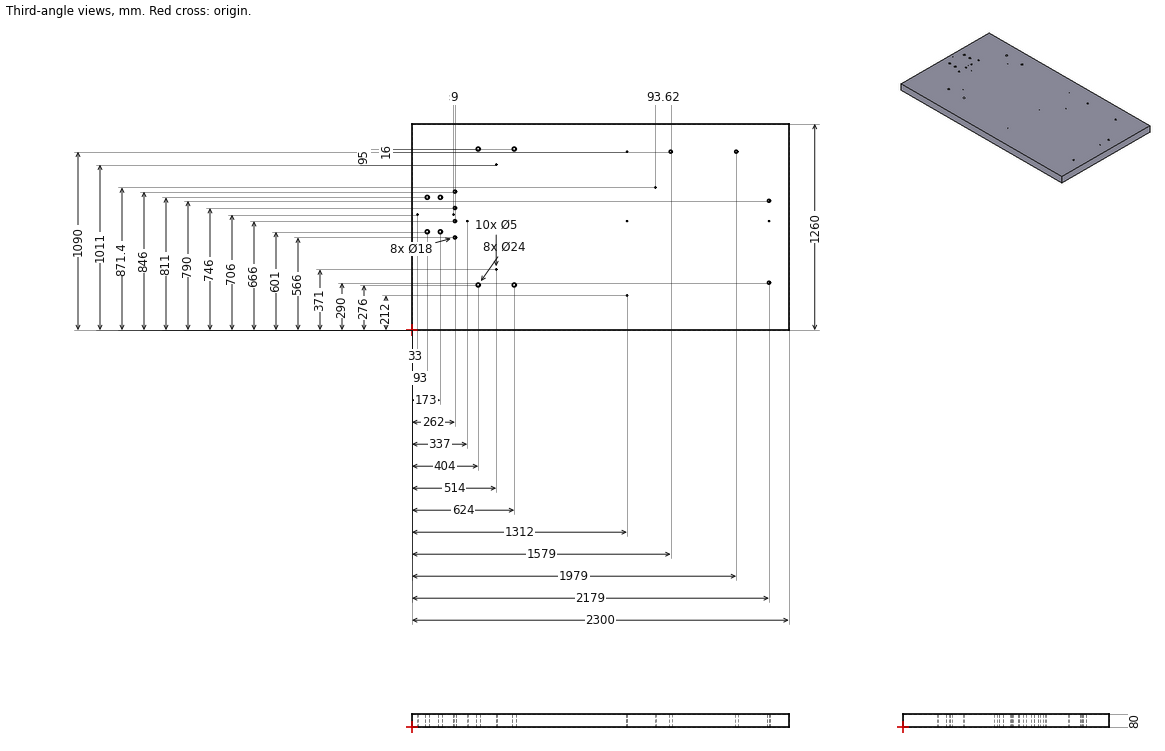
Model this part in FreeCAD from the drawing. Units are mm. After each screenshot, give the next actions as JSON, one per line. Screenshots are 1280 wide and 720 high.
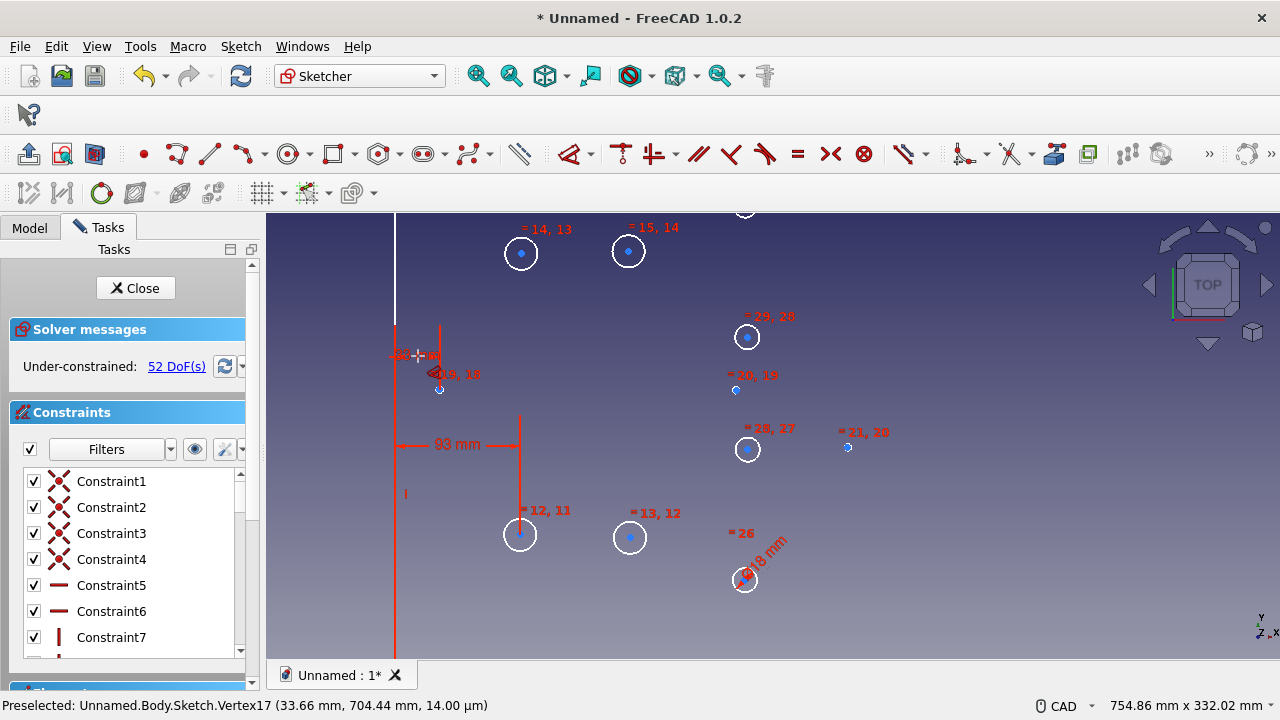
{"action": "scroll", "coordinate": [460, 425], "scroll_direction": "down", "scroll_amount": 9}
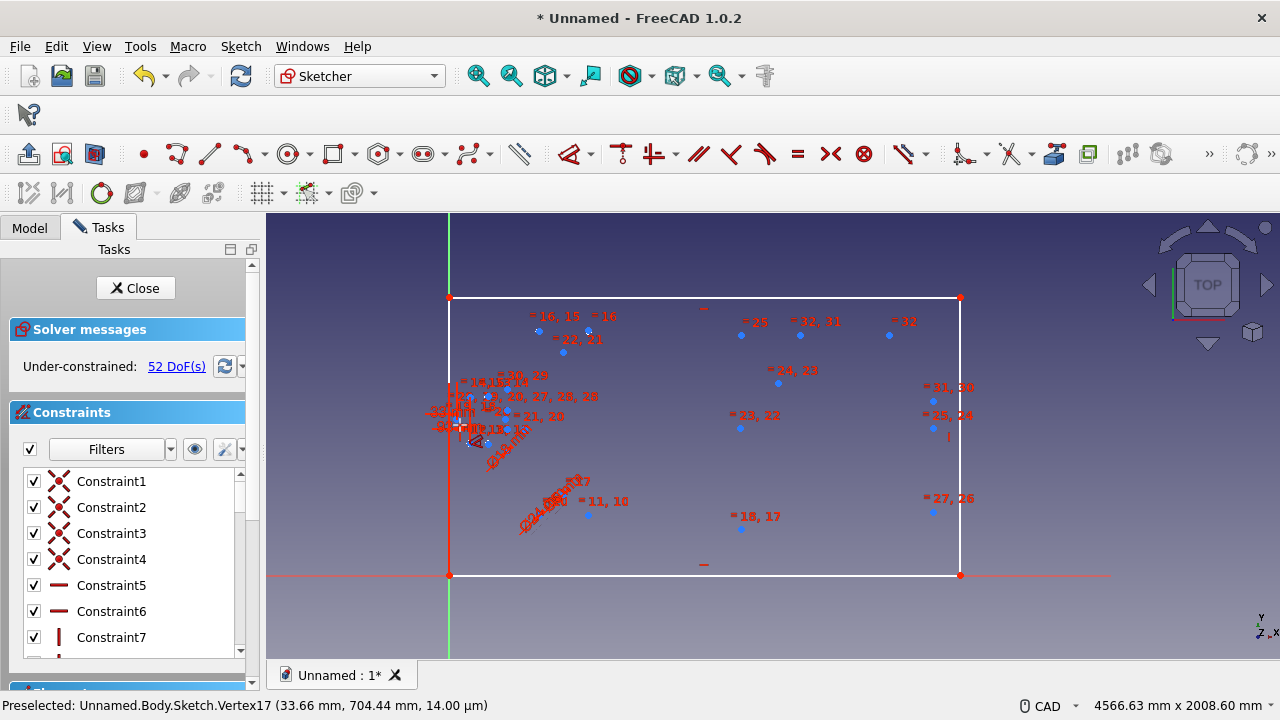
{"action": "scroll", "coordinate": [470, 397], "scroll_direction": "up", "scroll_amount": 4}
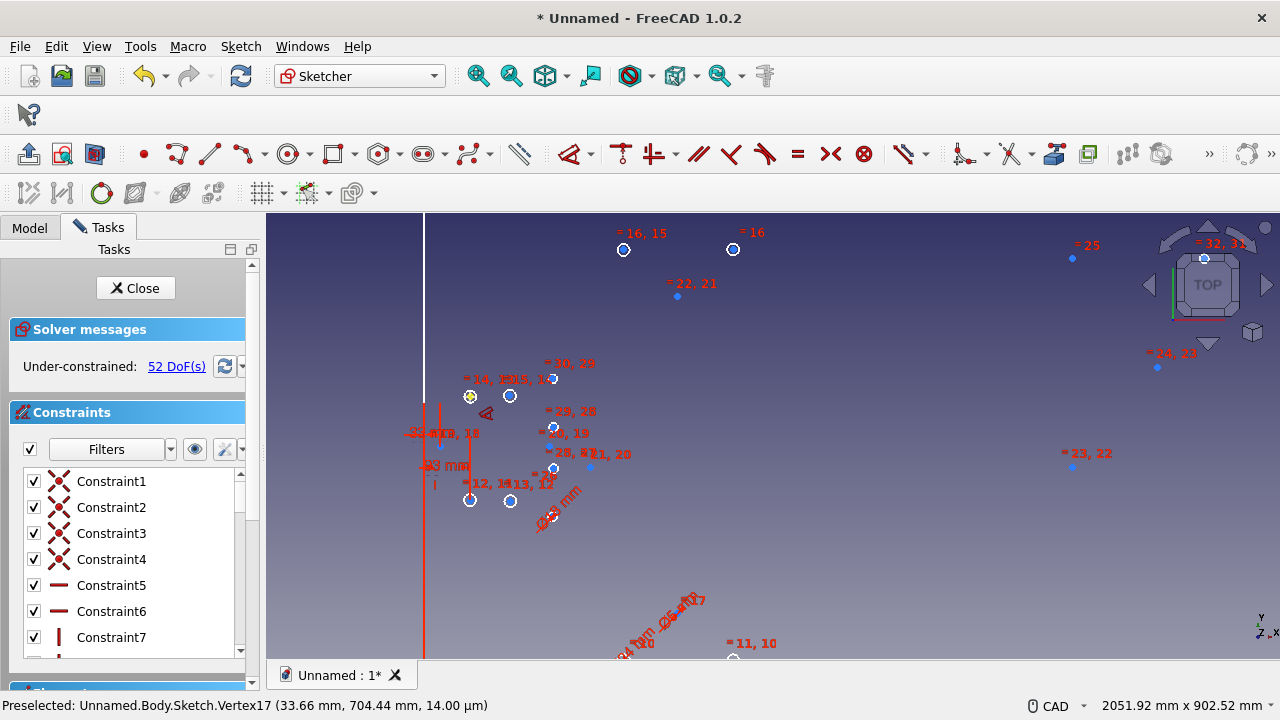
{"action": "left_click", "coordinate": [470, 397]}
{"action": "left_click", "coordinate": [447, 363]}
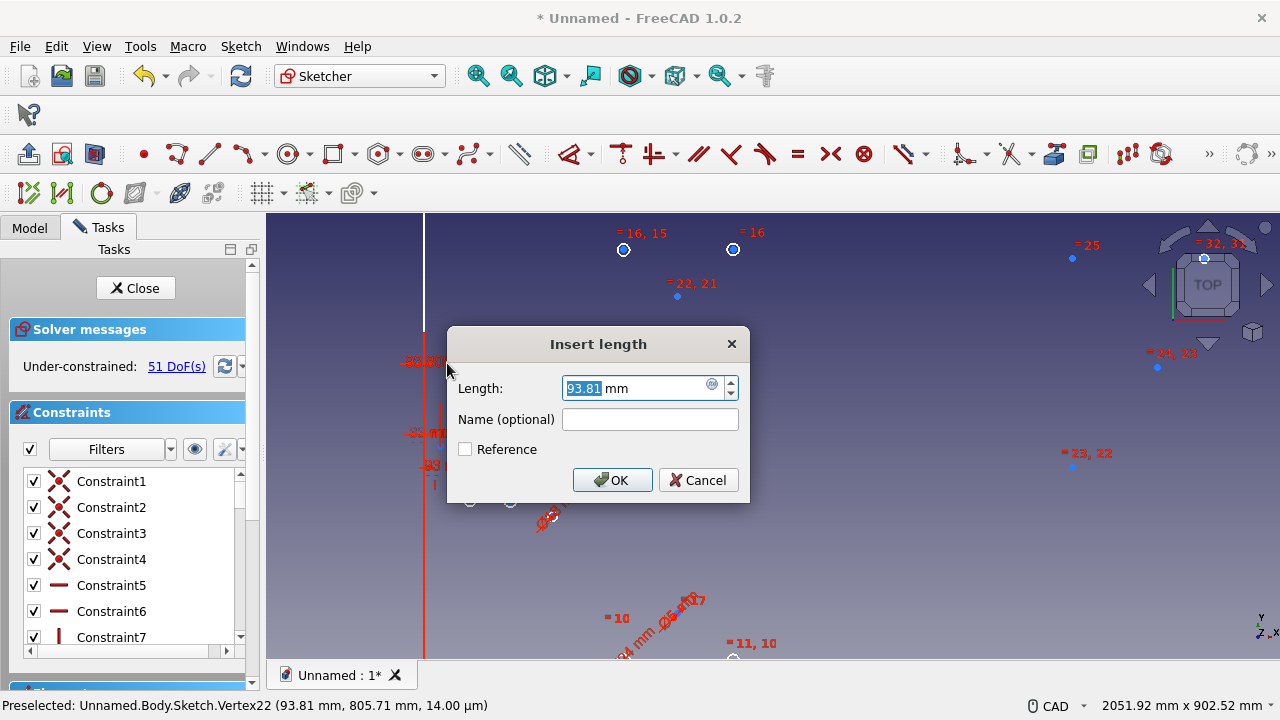
{"action": "type", "text": "93"}
{"action": "key", "text": "Return"}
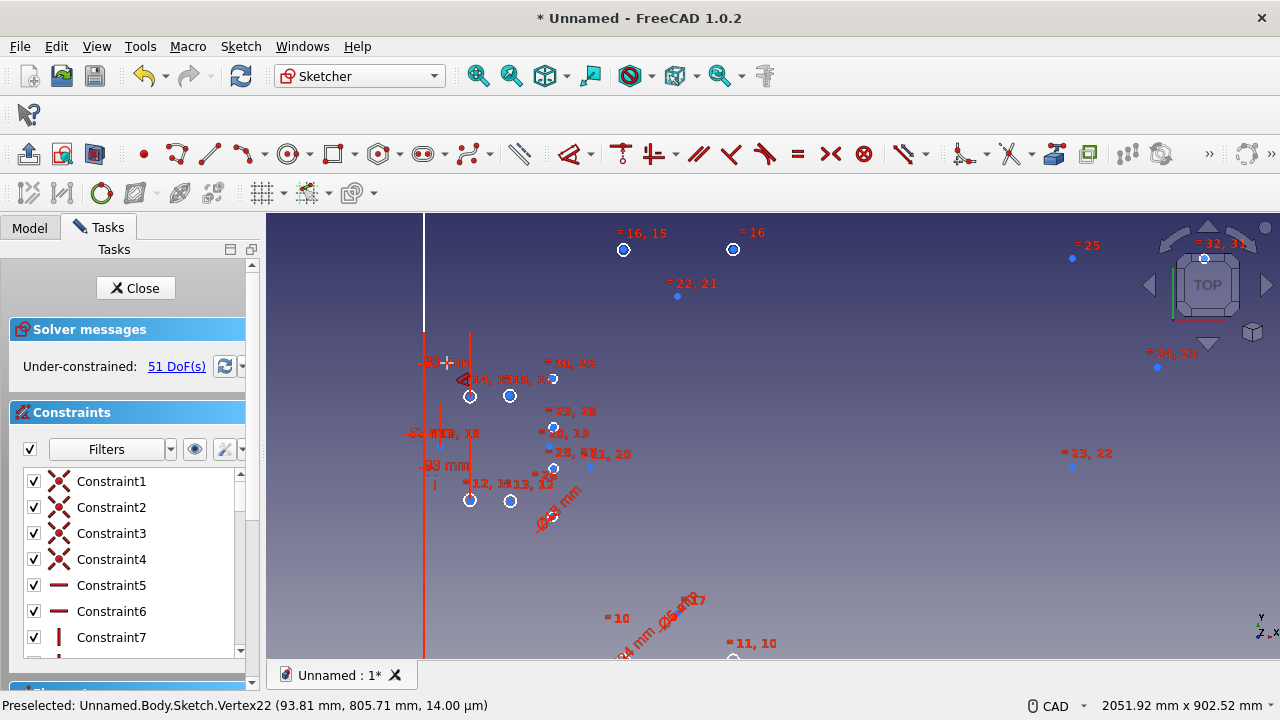
{"action": "scroll", "coordinate": [554, 469], "scroll_direction": "up", "scroll_amount": 11}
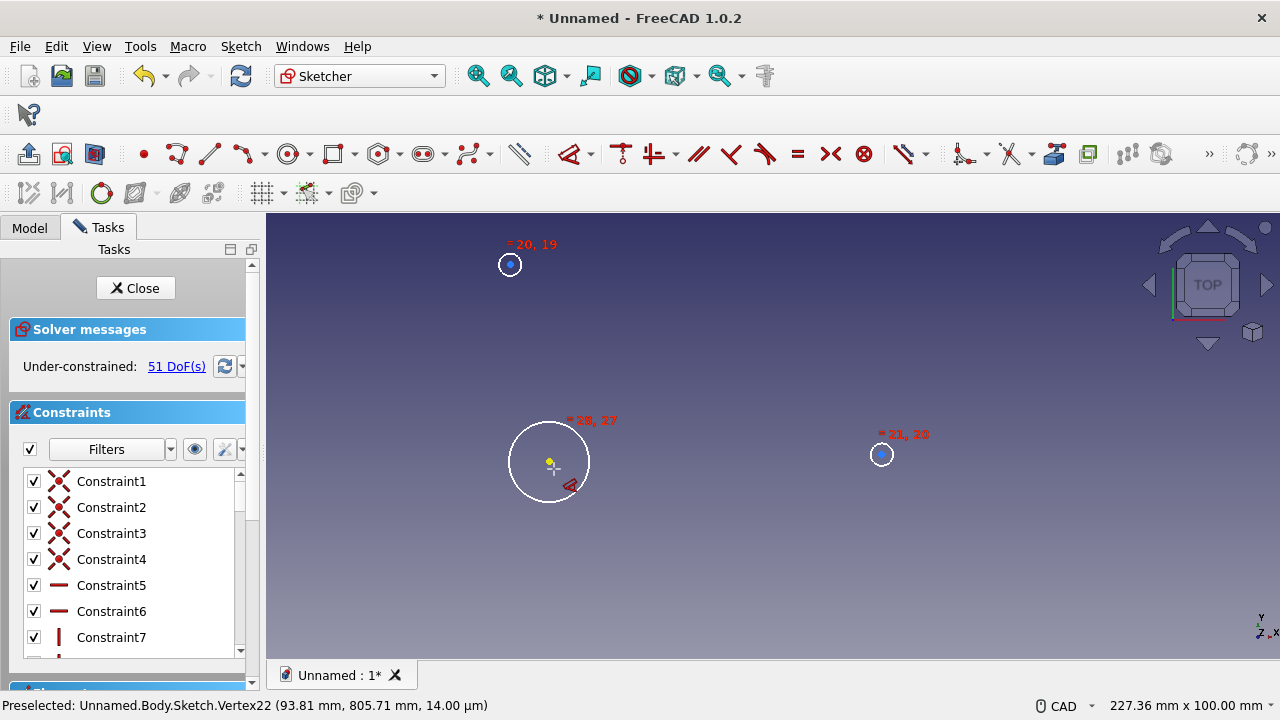
{"action": "left_click", "coordinate": [549, 462]}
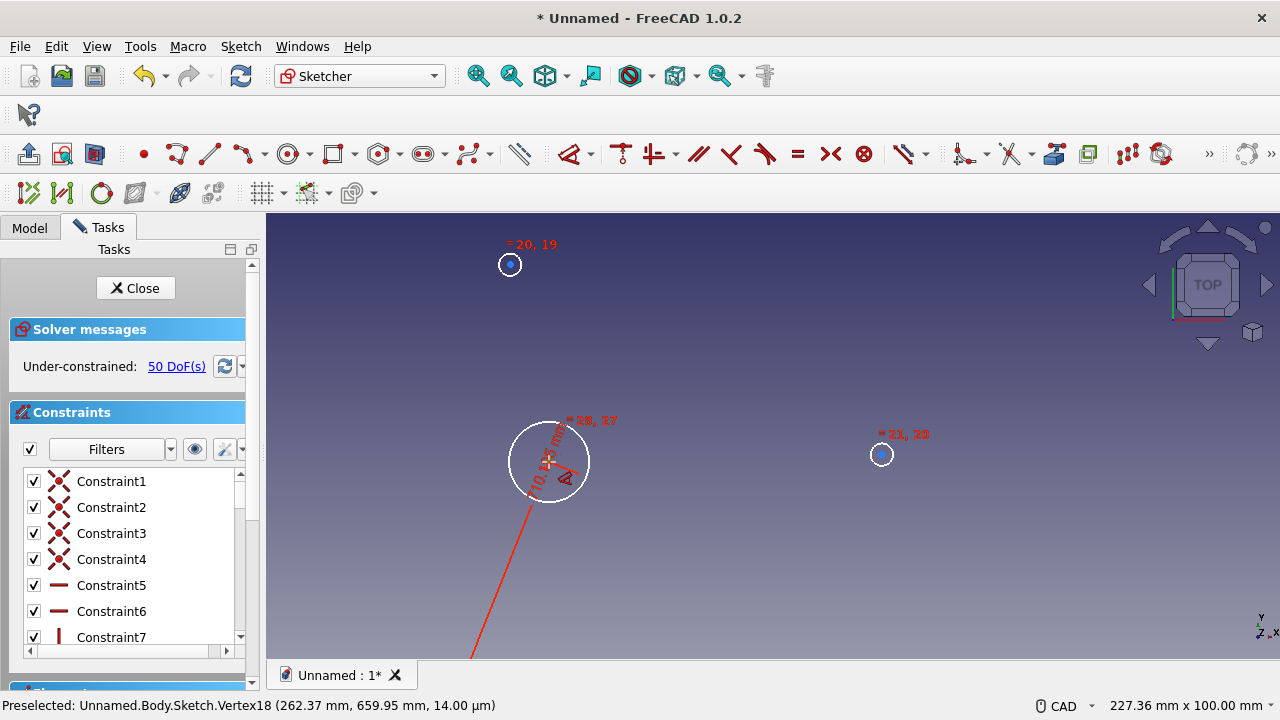
{"action": "left_click", "coordinate": [510, 265]}
{"action": "left_click", "coordinate": [530, 520]}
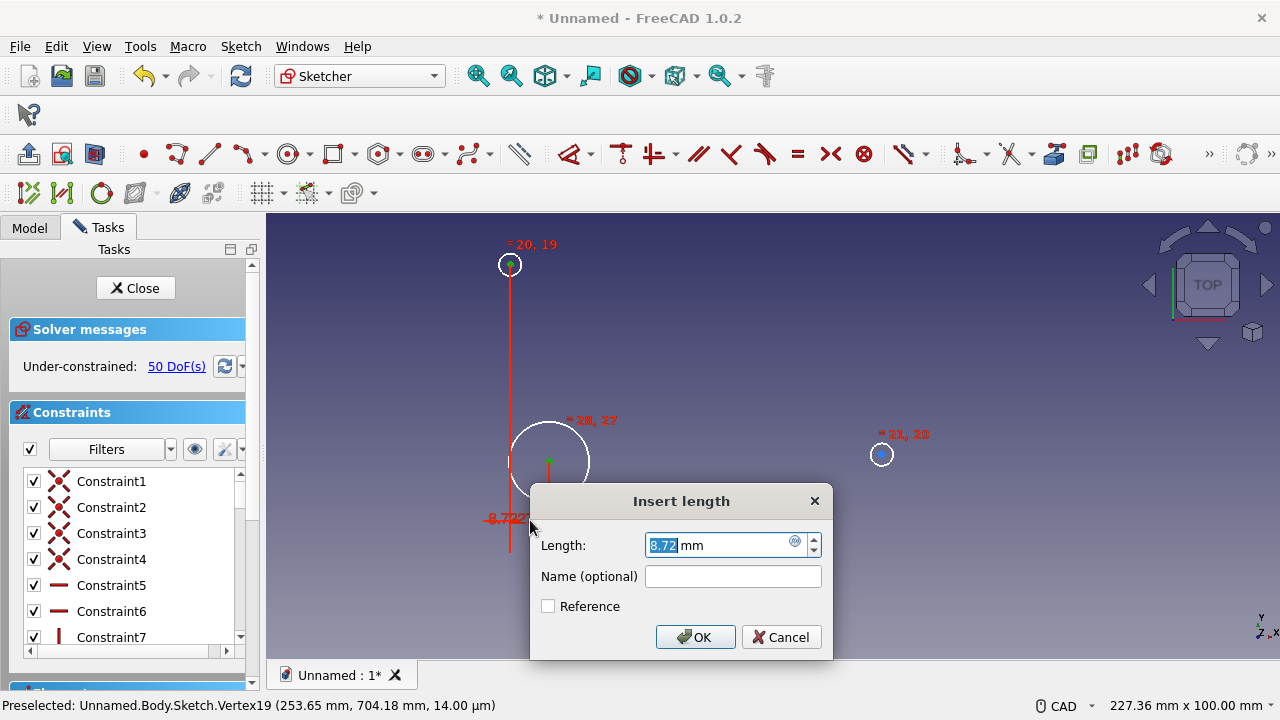
{"action": "type", "text": "9"}
{"action": "key", "text": "Return"}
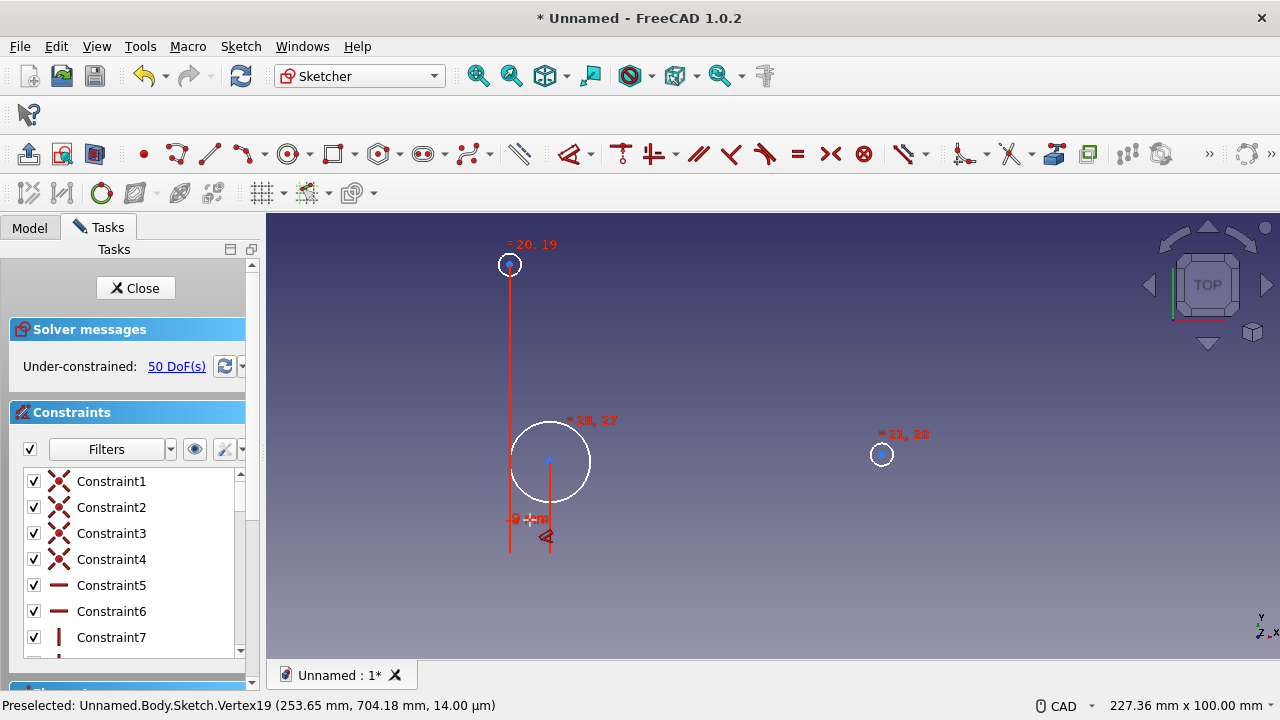
{"action": "scroll", "coordinate": [505, 428], "scroll_direction": "down", "scroll_amount": 15}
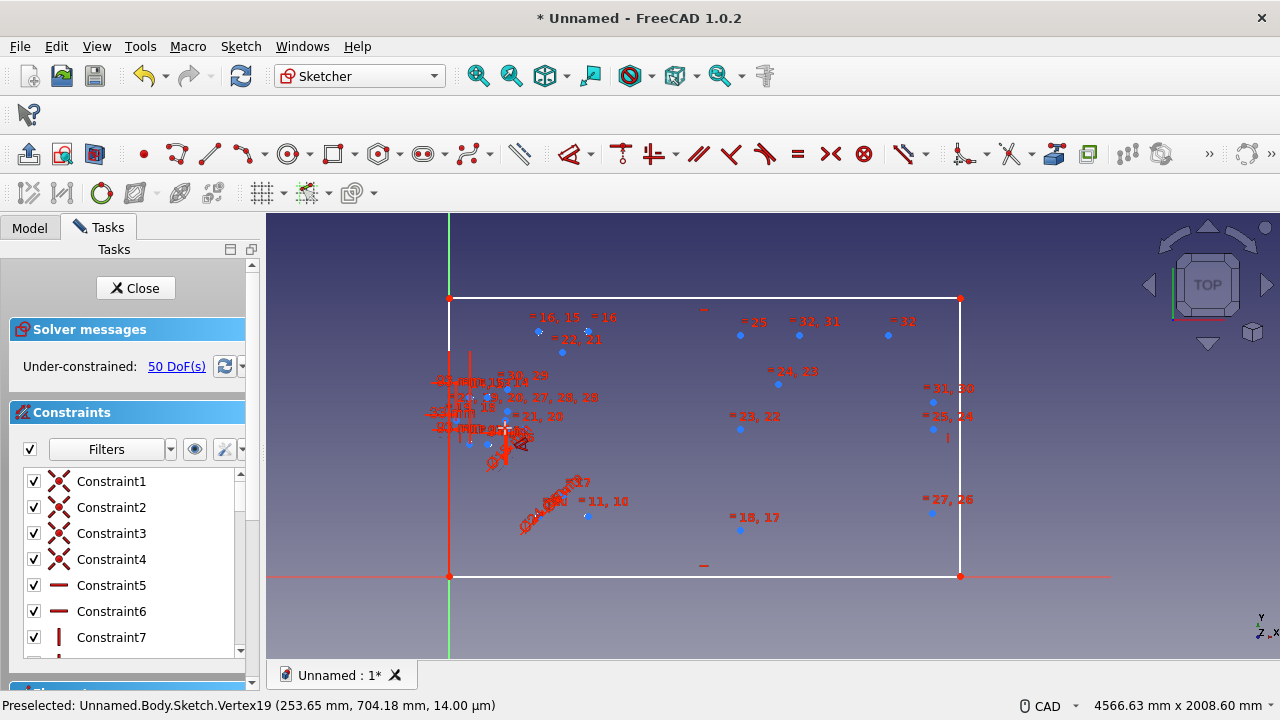
{"action": "scroll", "coordinate": [507, 452], "scroll_direction": "up", "scroll_amount": 15}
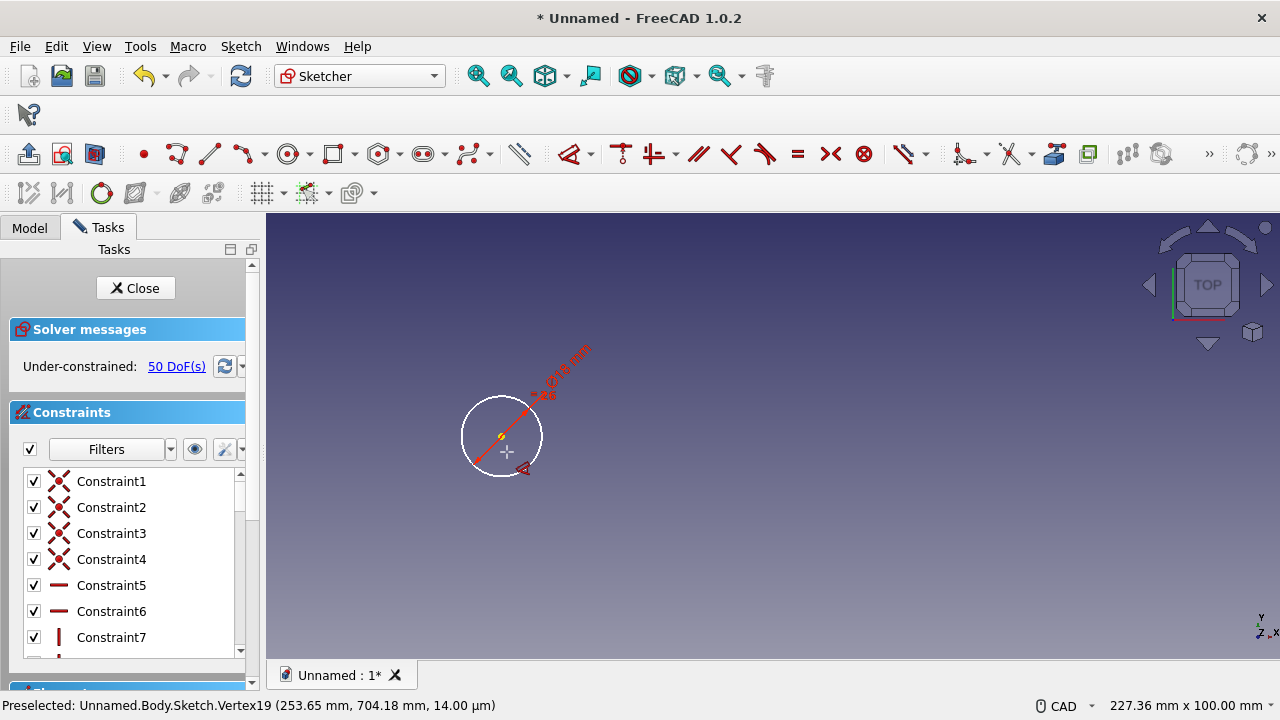
{"action": "left_click", "coordinate": [502, 436]}